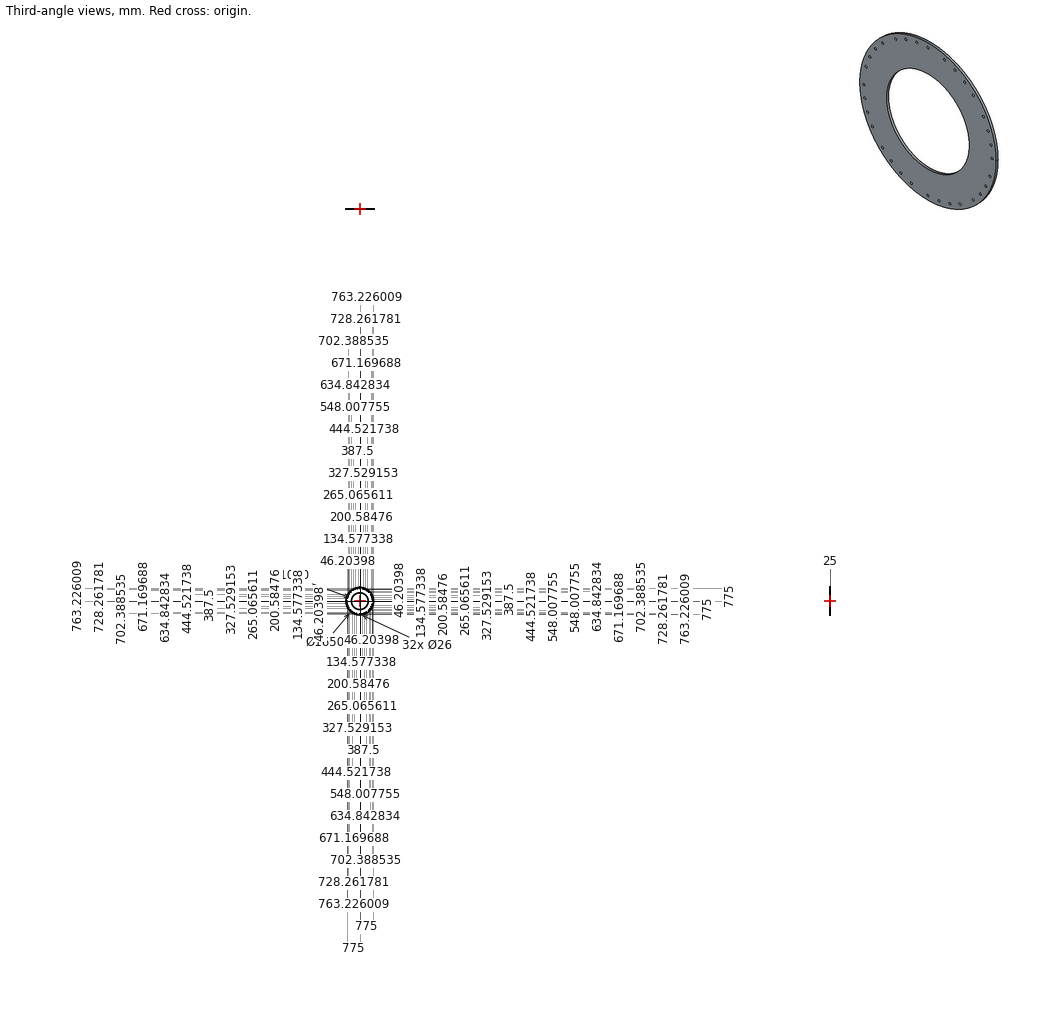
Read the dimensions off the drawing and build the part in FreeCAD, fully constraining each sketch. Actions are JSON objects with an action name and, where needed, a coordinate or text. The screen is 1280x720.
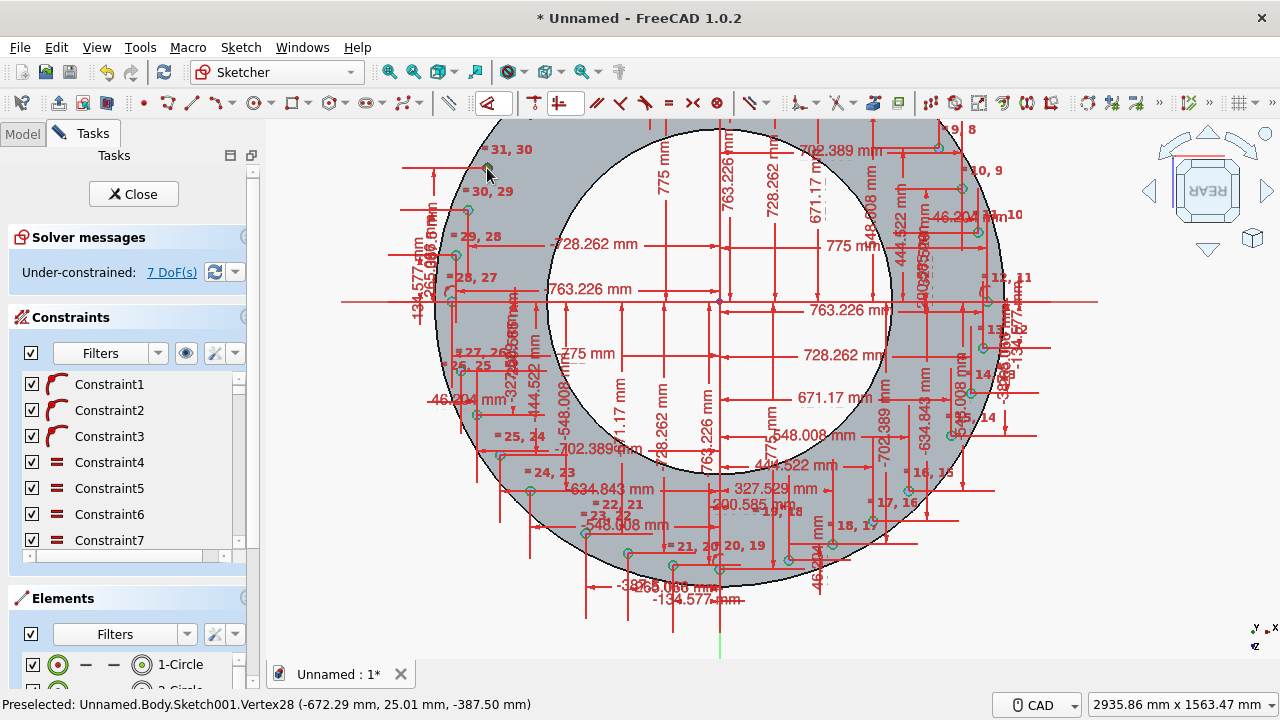
{"action": "key", "text": "l"}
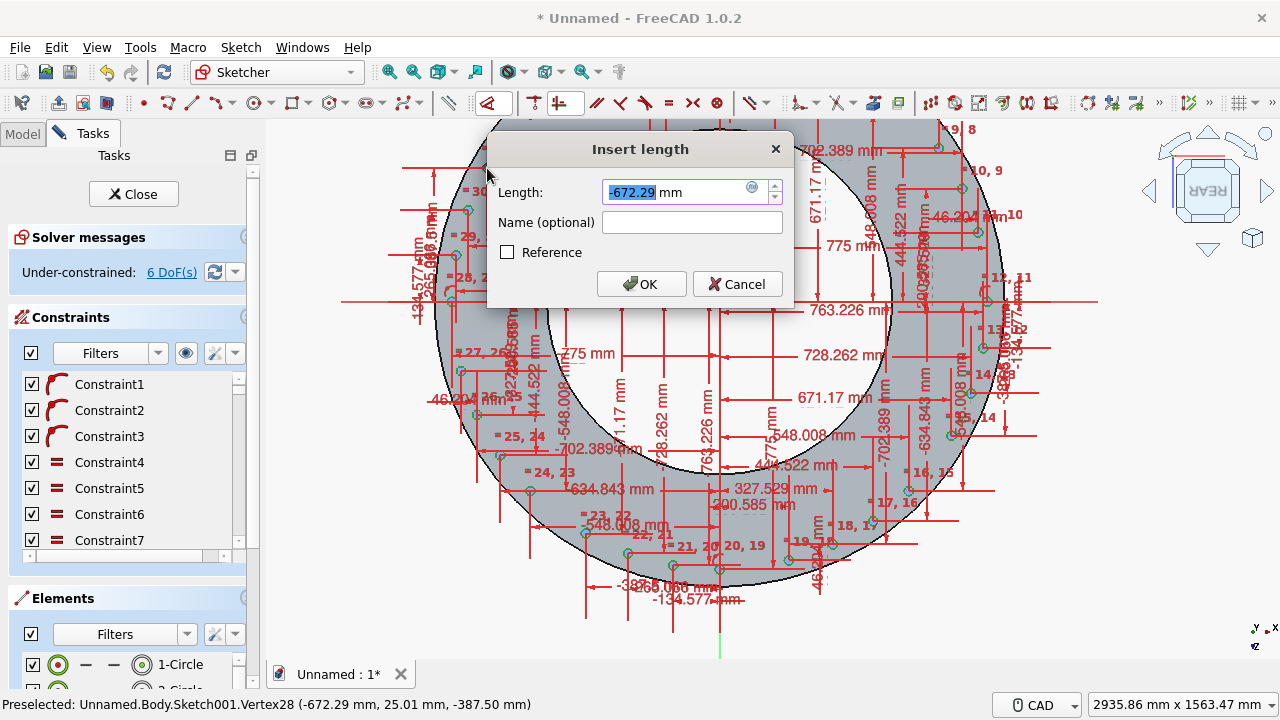
{"action": "type", "text": "-671.169688"}
{"action": "key", "text": "Return"}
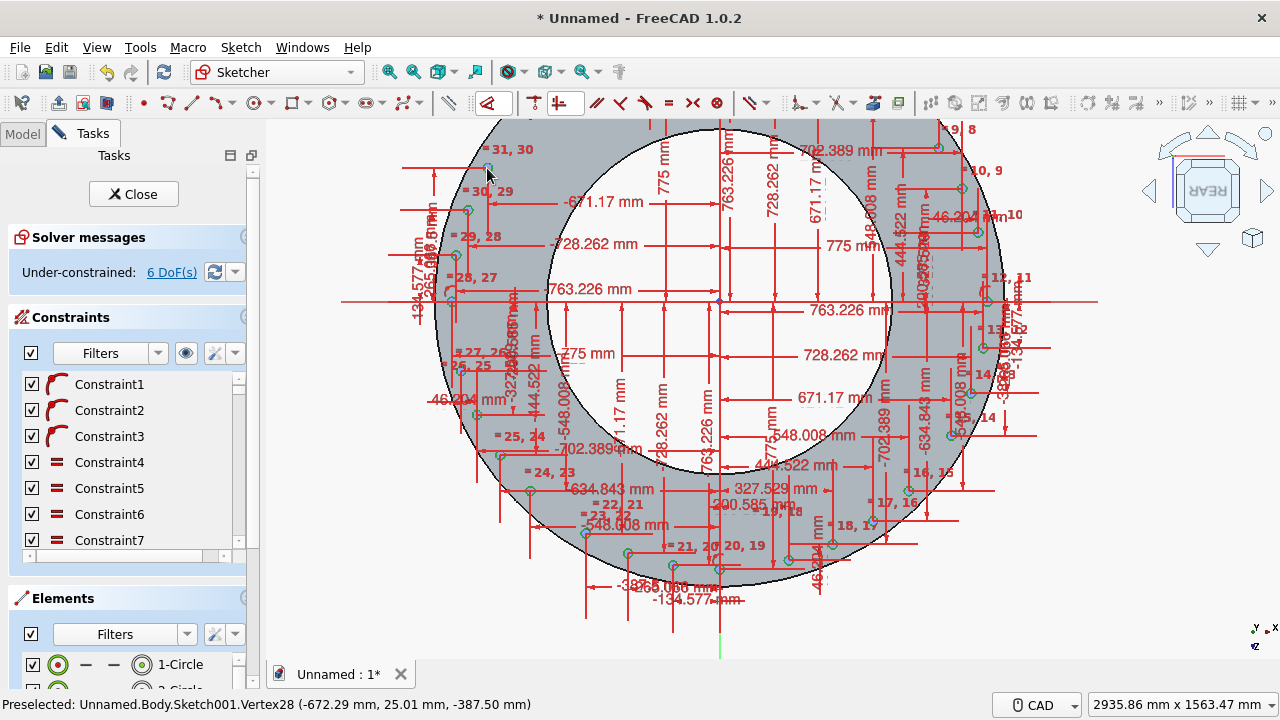
{"action": "scroll", "coordinate": [674, 566], "scroll_direction": "down", "scroll_amount": 2}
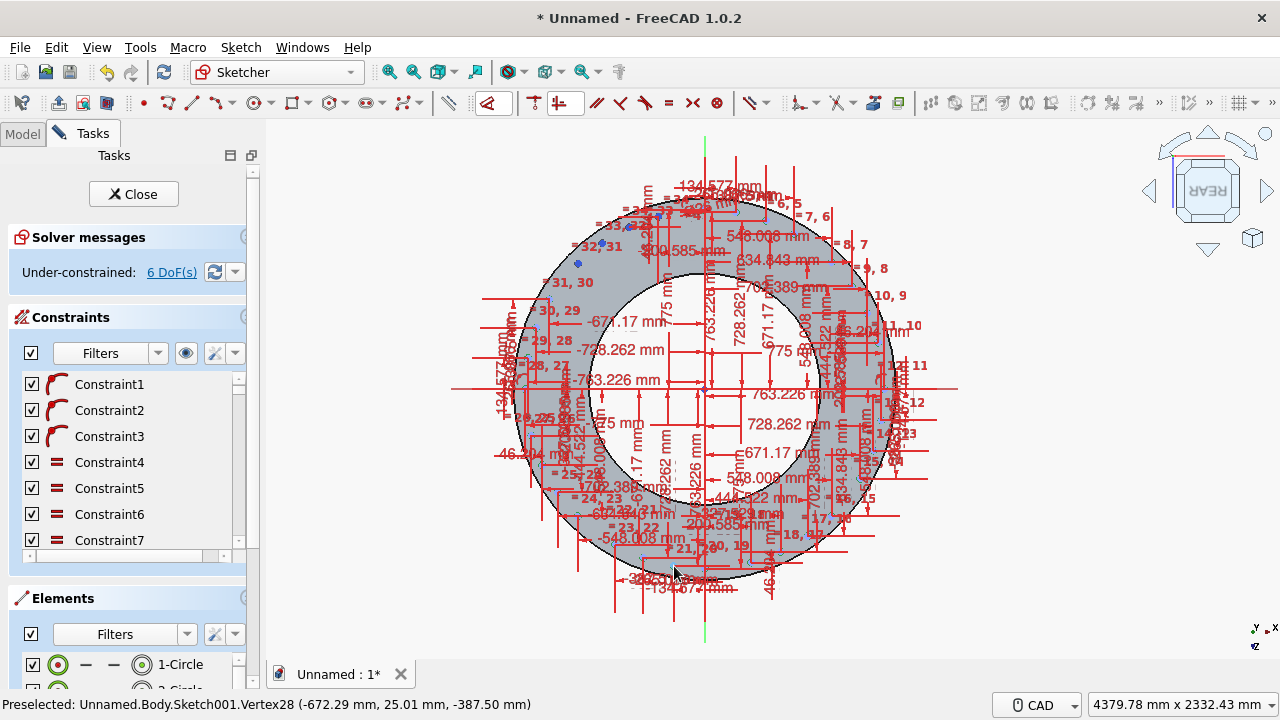
{"action": "left_click", "coordinate": [578, 264]}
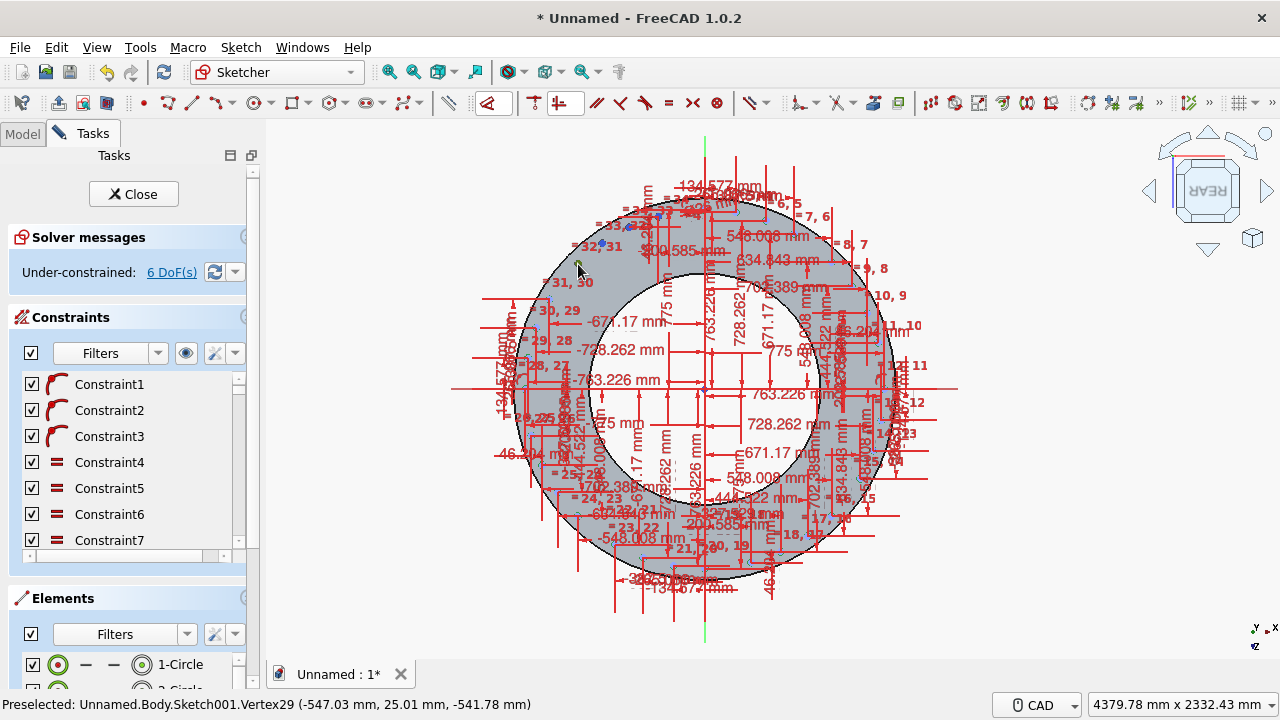
{"action": "key", "text": "l"}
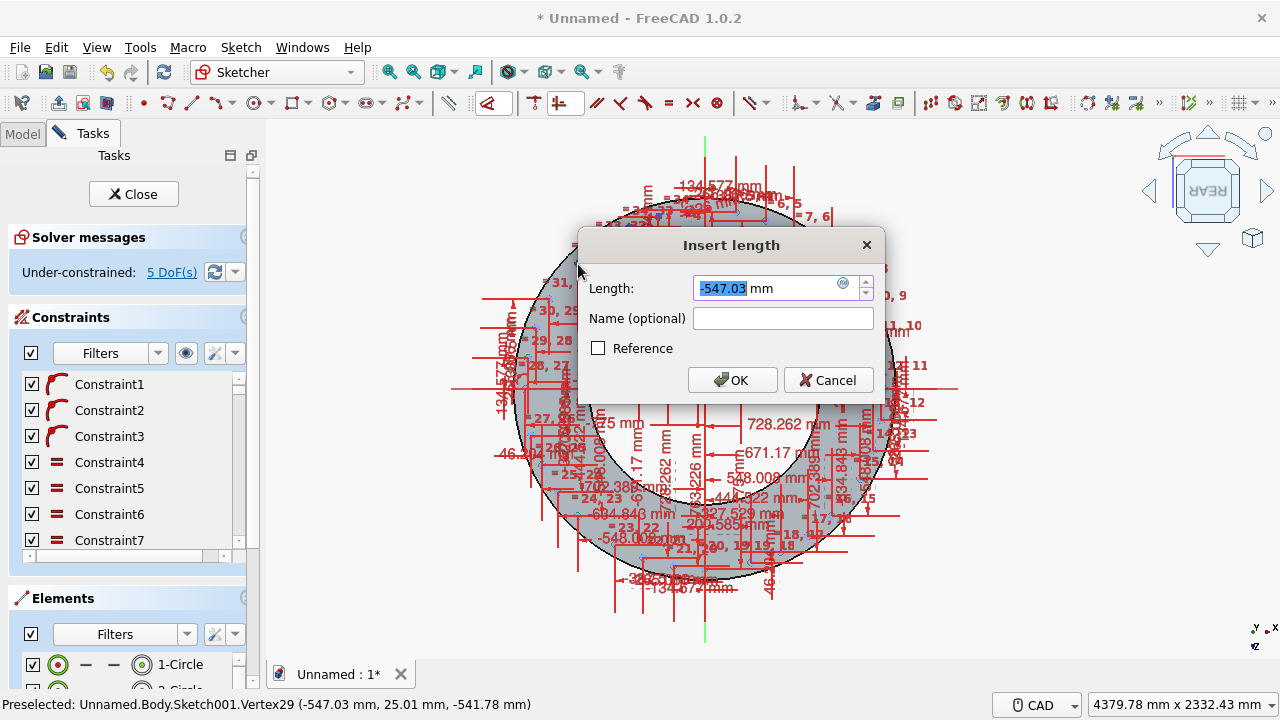
{"action": "type", "text": "-548.007755"}
{"action": "key", "text": "Return"}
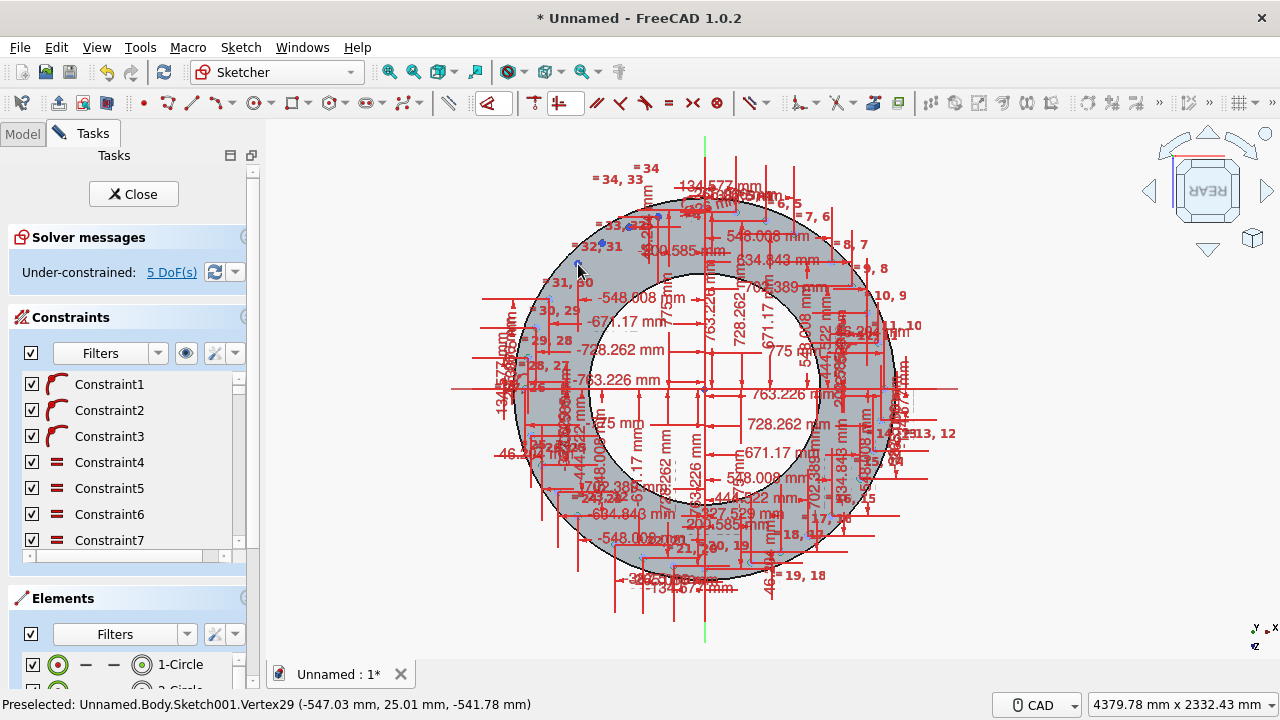
{"action": "left_click", "coordinate": [578, 264]}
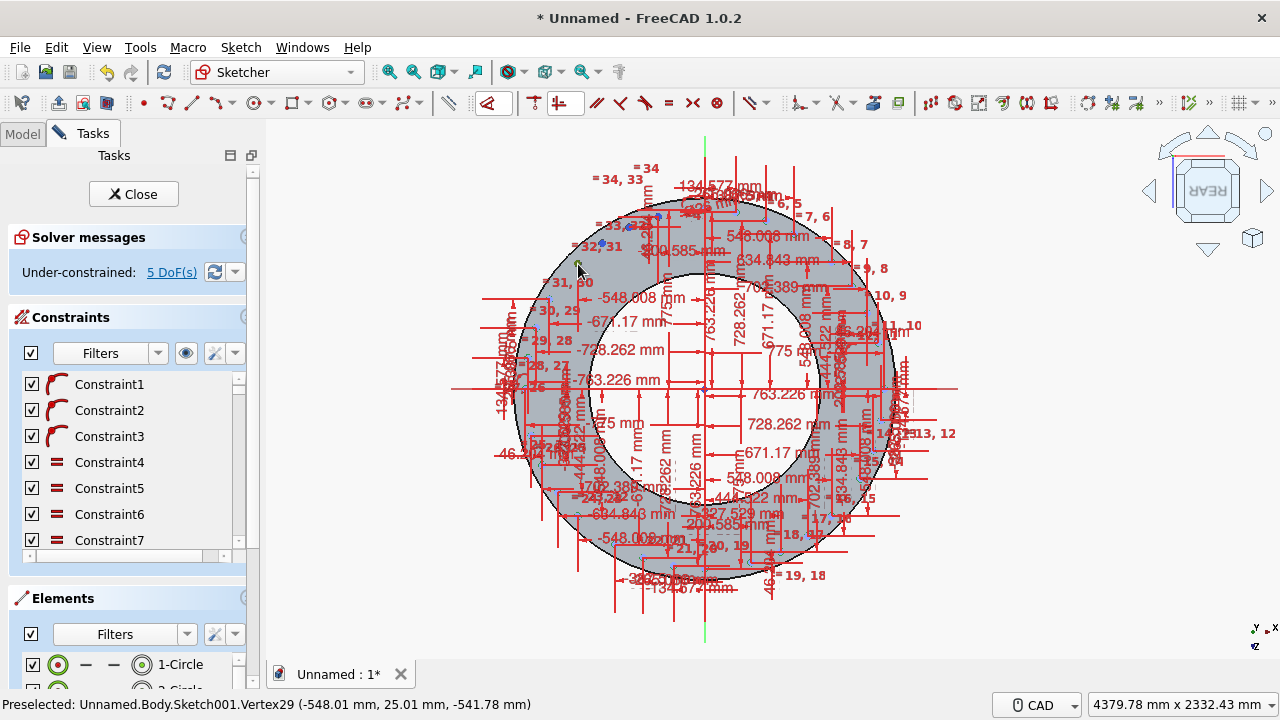
{"action": "key", "text": "i"}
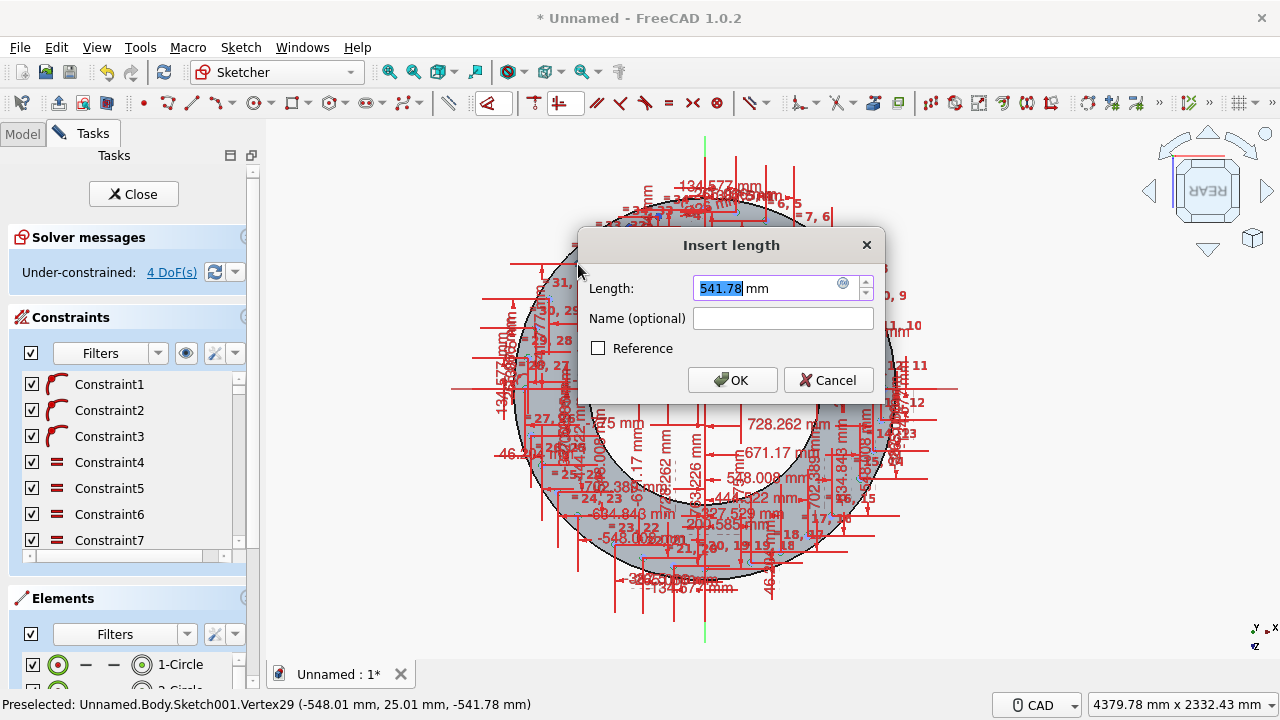
{"action": "type", "text": "548.007755"}
{"action": "key", "text": "Return"}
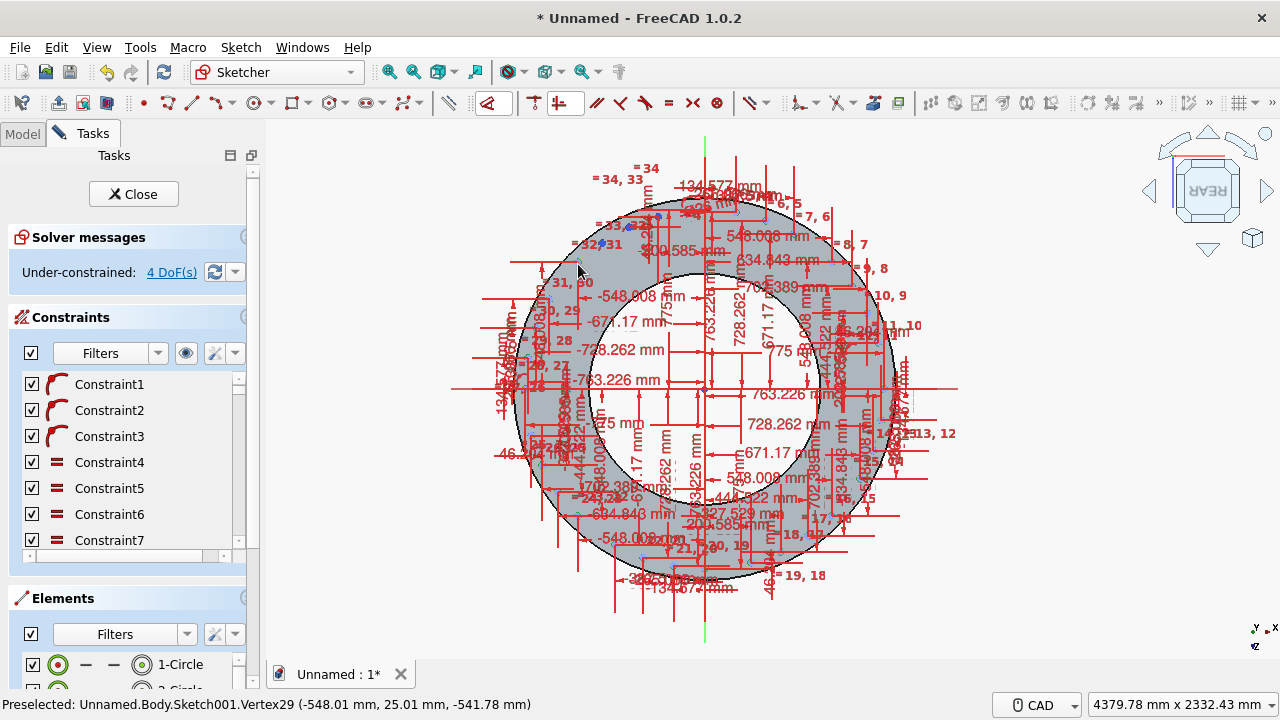
{"action": "left_click", "coordinate": [602, 243]}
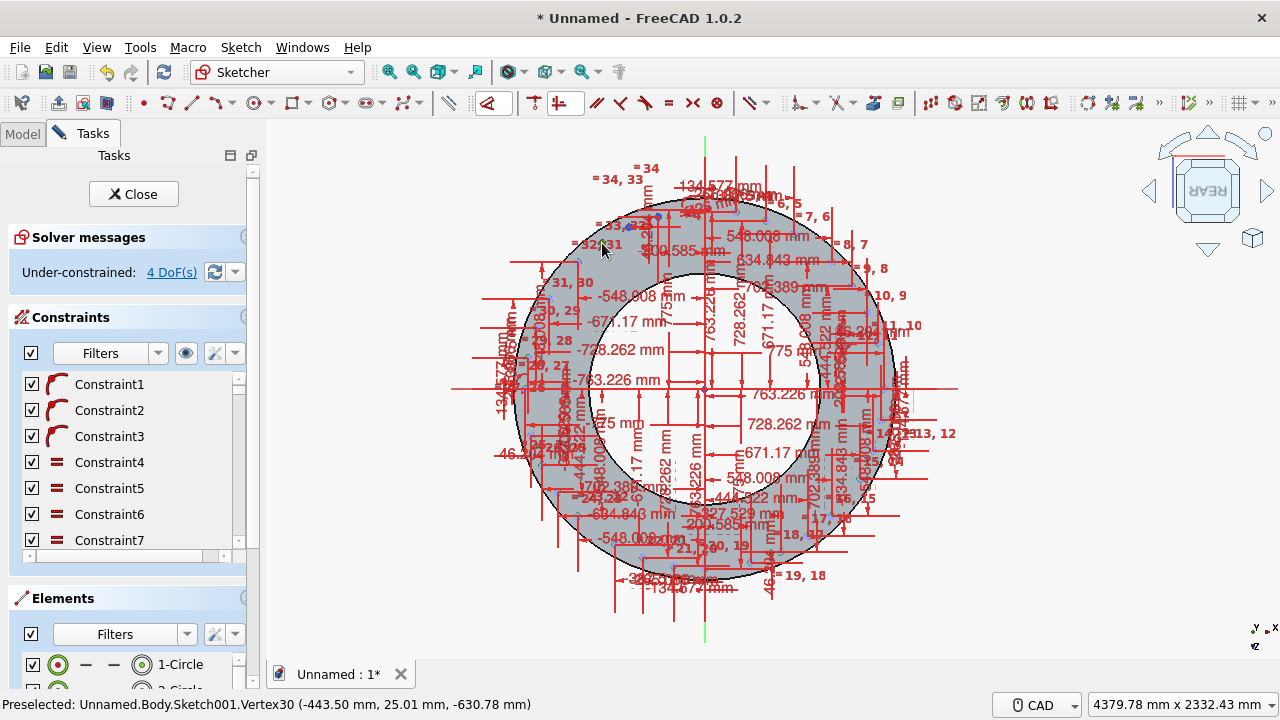
{"action": "key", "text": "l"}